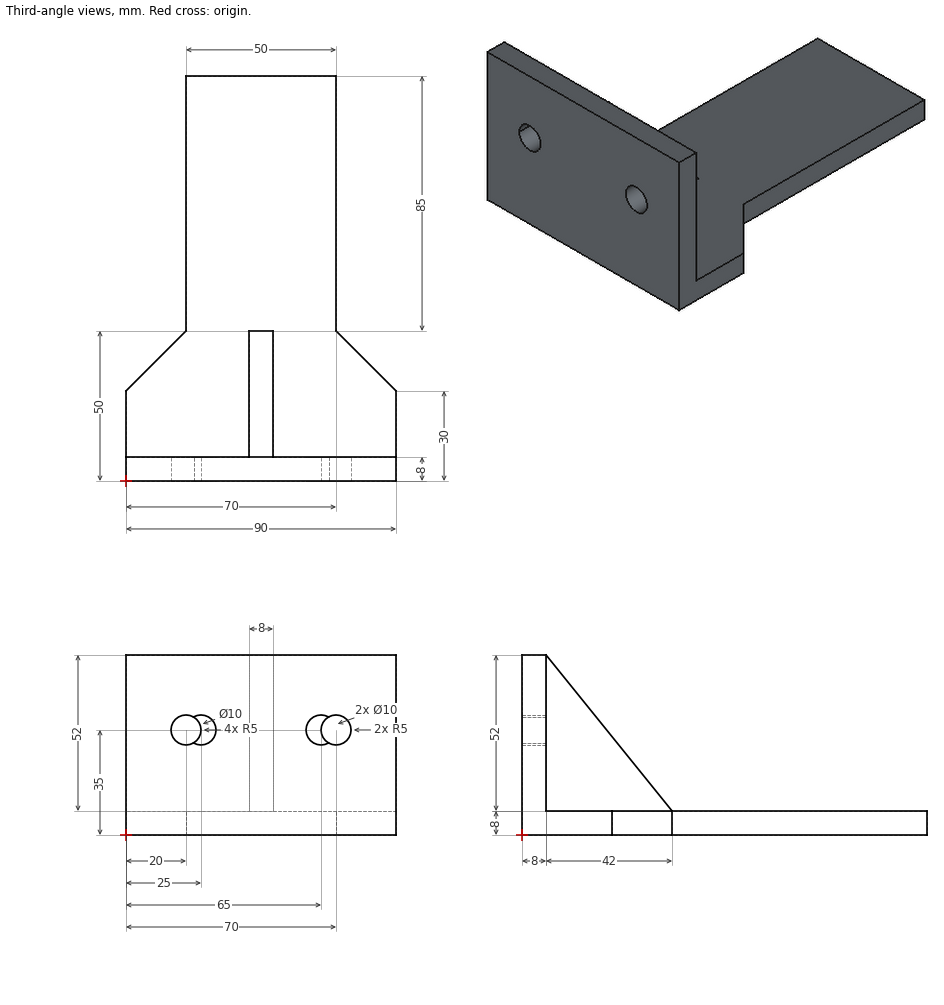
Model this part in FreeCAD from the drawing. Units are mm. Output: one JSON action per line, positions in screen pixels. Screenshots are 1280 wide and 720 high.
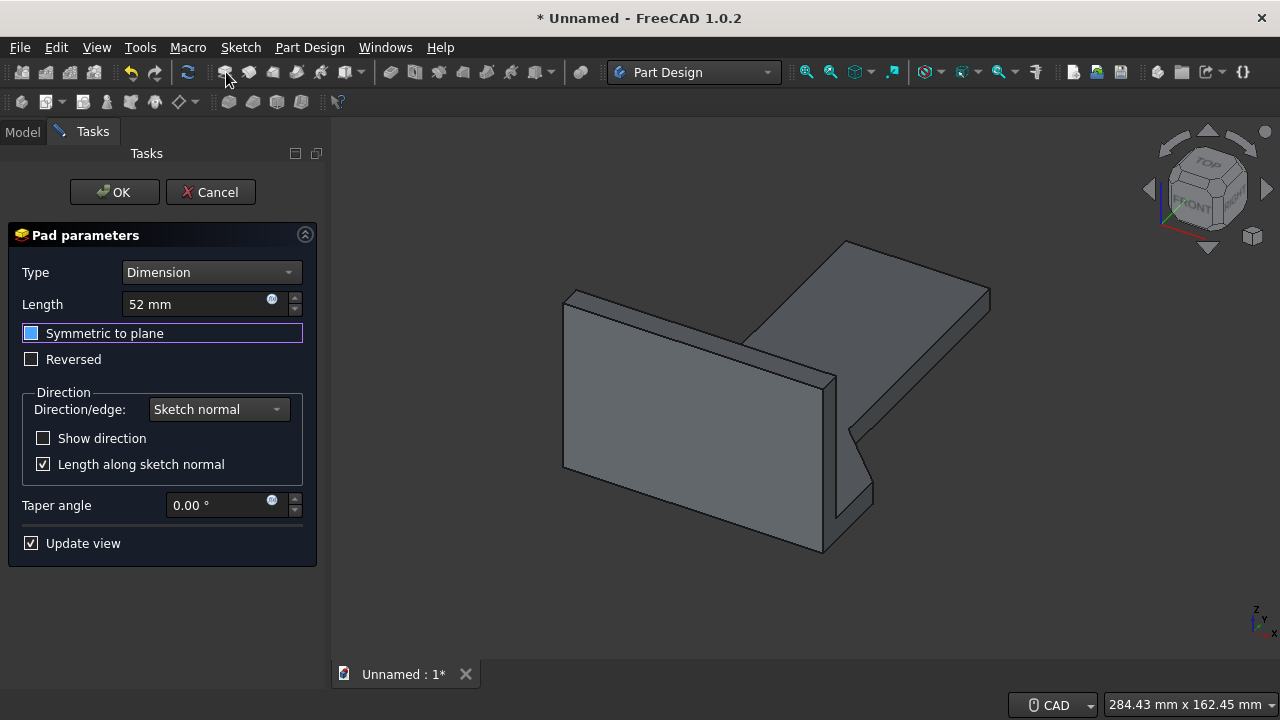
{"action": "left_click", "coordinate": [115, 192]}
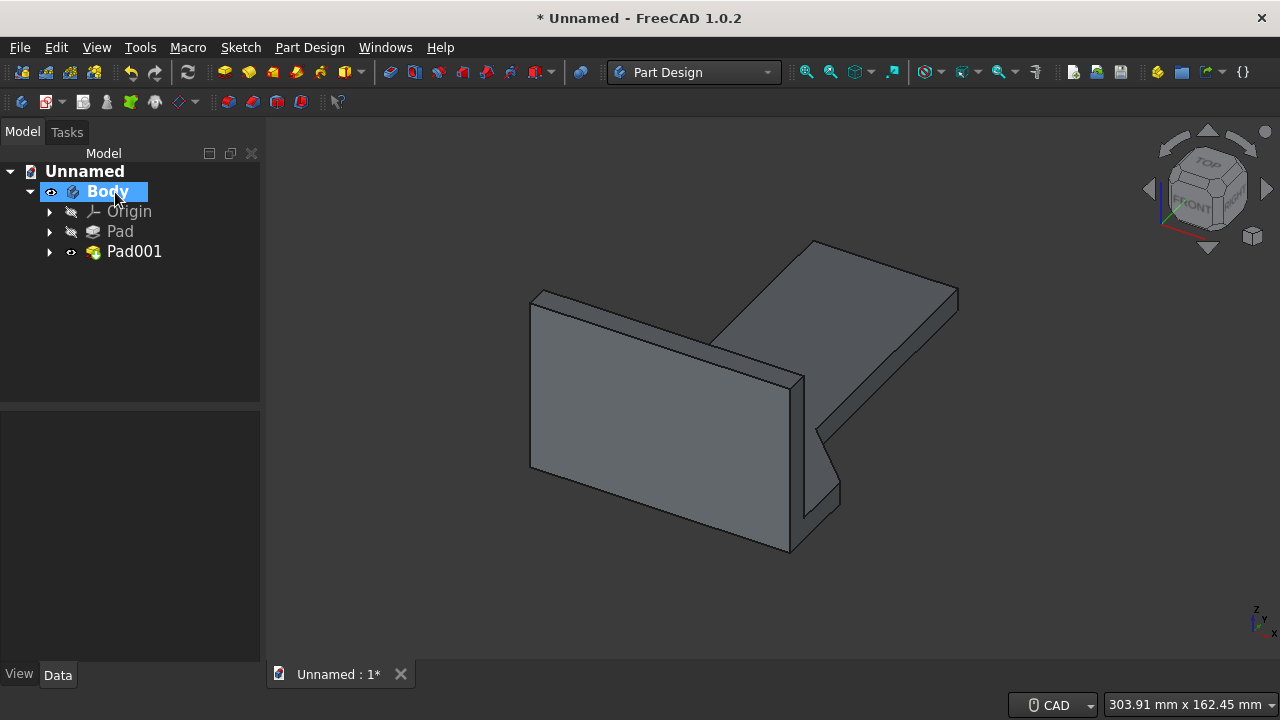
{"action": "left_click", "coordinate": [808, 72]}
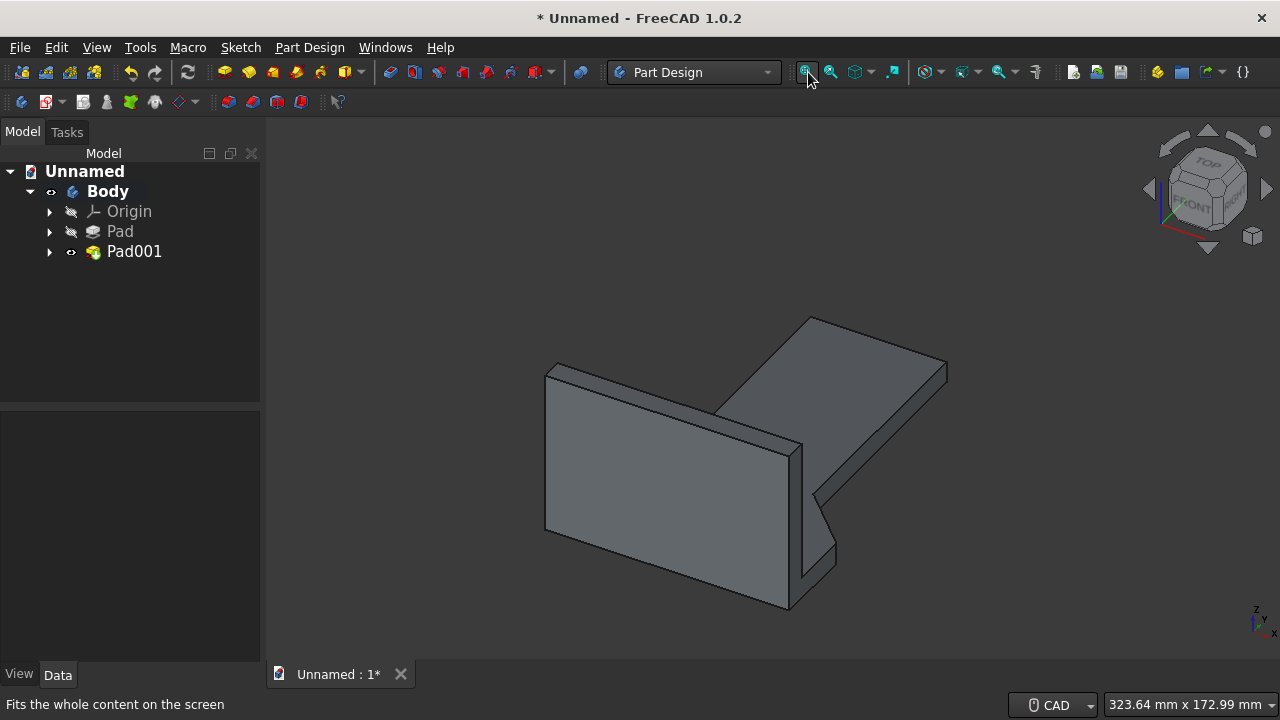
{"action": "left_click", "coordinate": [50, 212]}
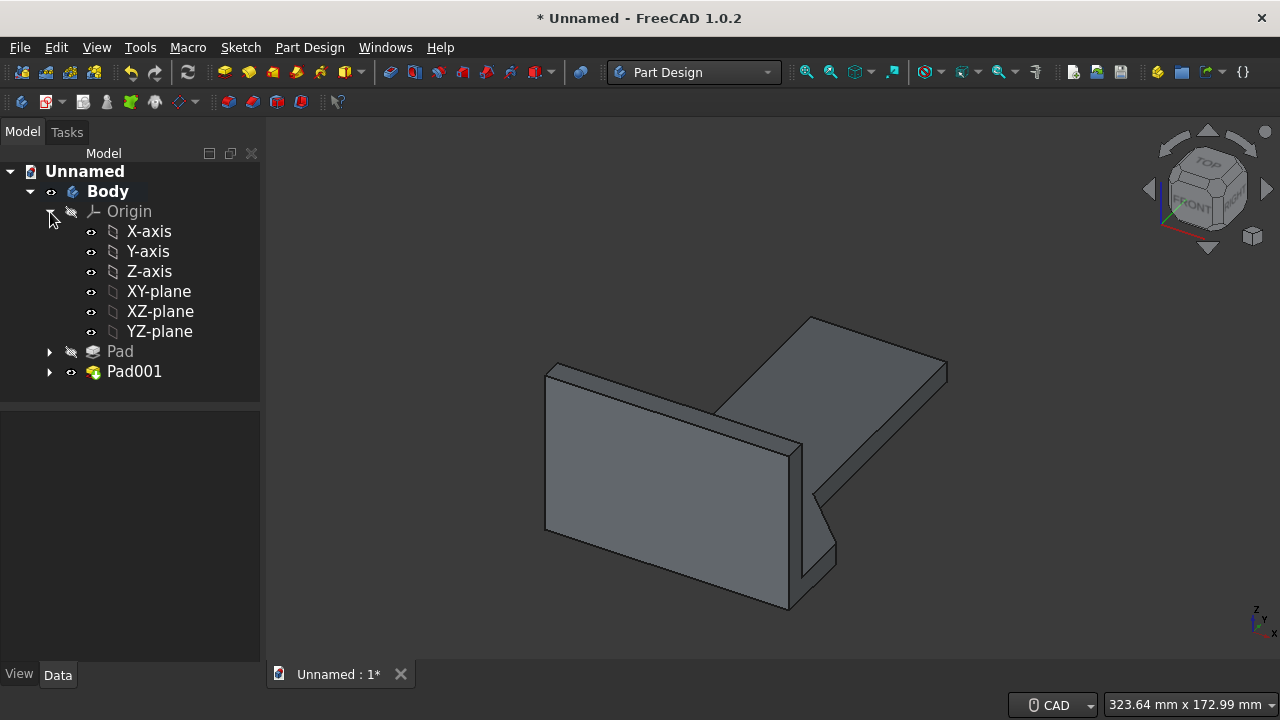
{"action": "left_click", "coordinate": [136, 332]}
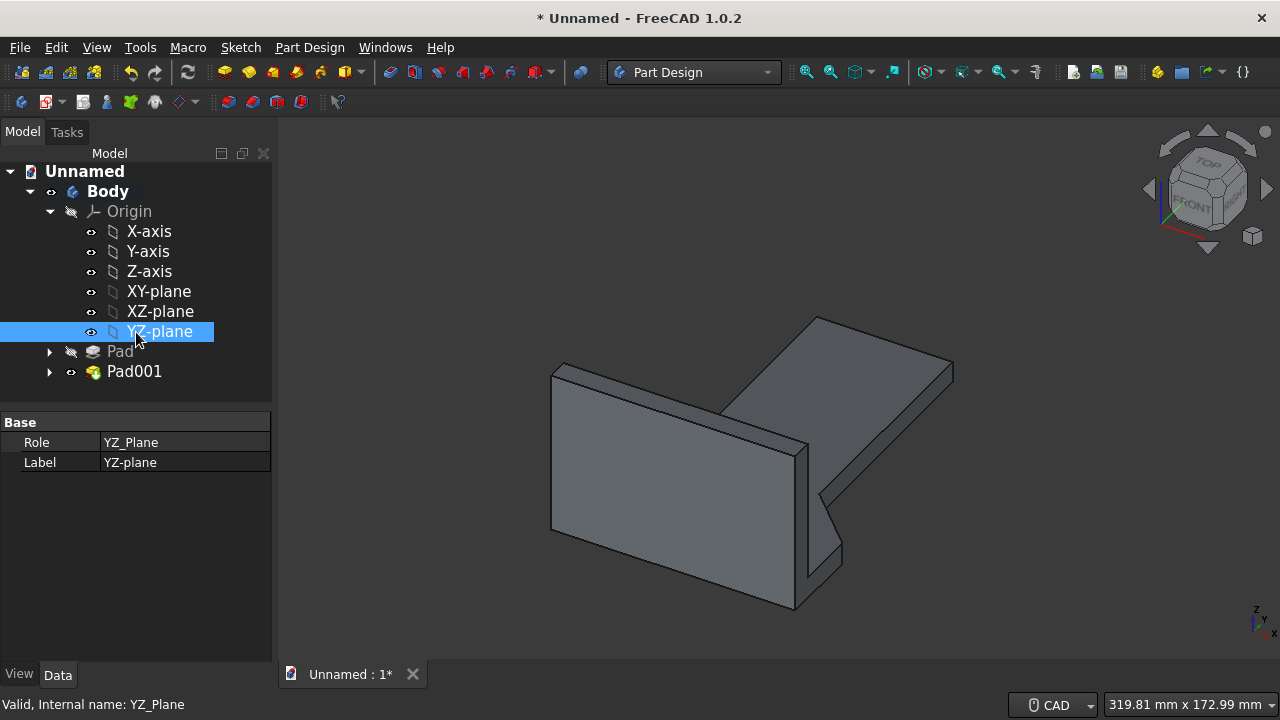
{"action": "left_click", "coordinate": [180, 102]}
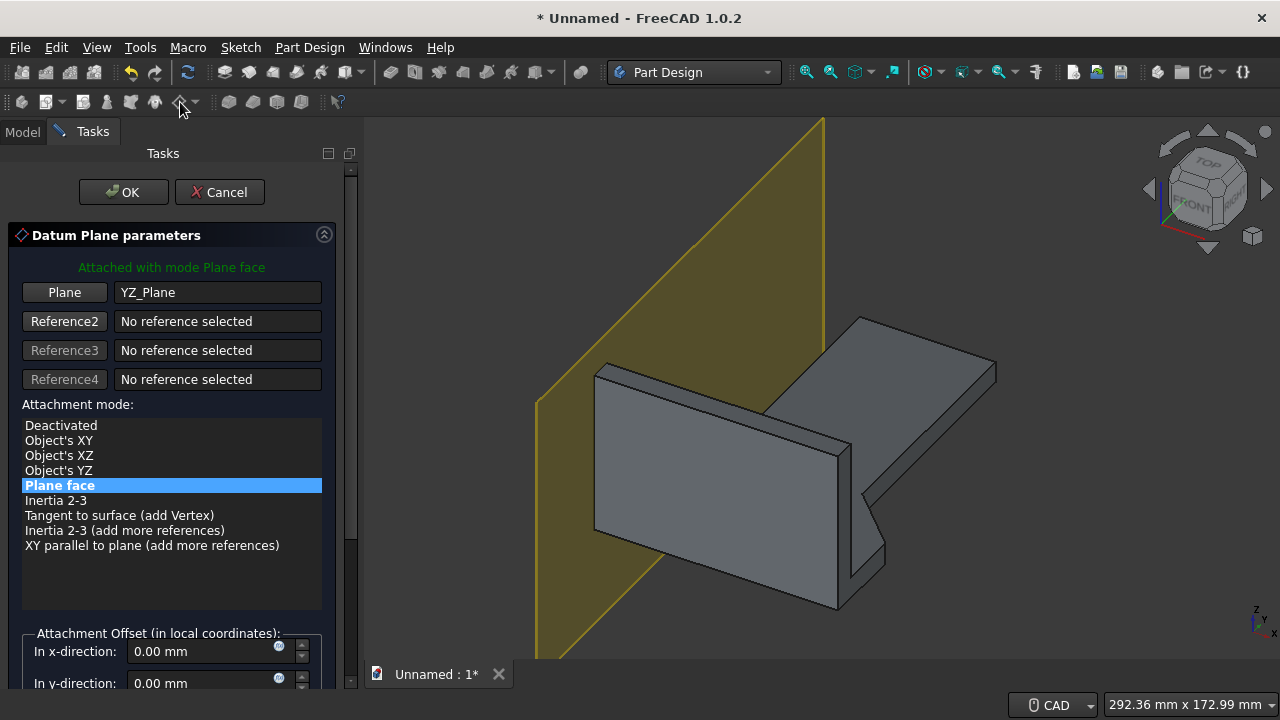
{"action": "scroll", "coordinate": [351, 426], "scroll_direction": "down", "scroll_amount": 2}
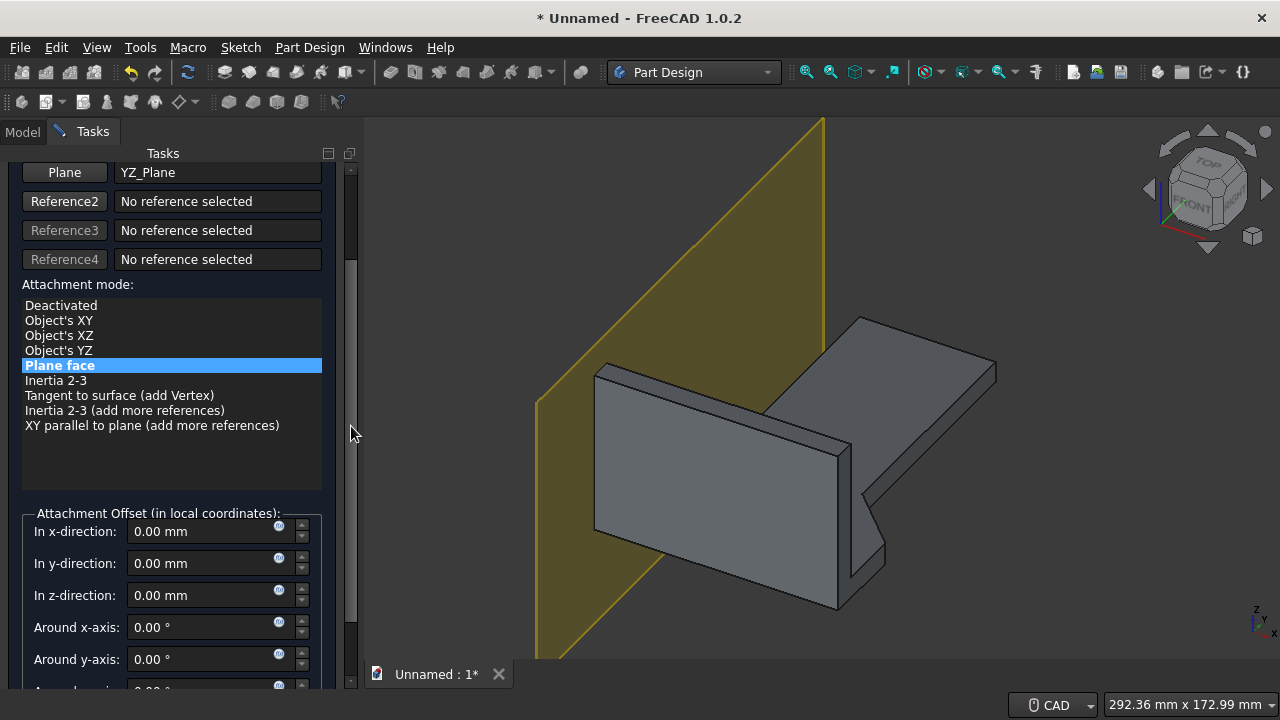
{"action": "triple_click", "coordinate": [210, 595]}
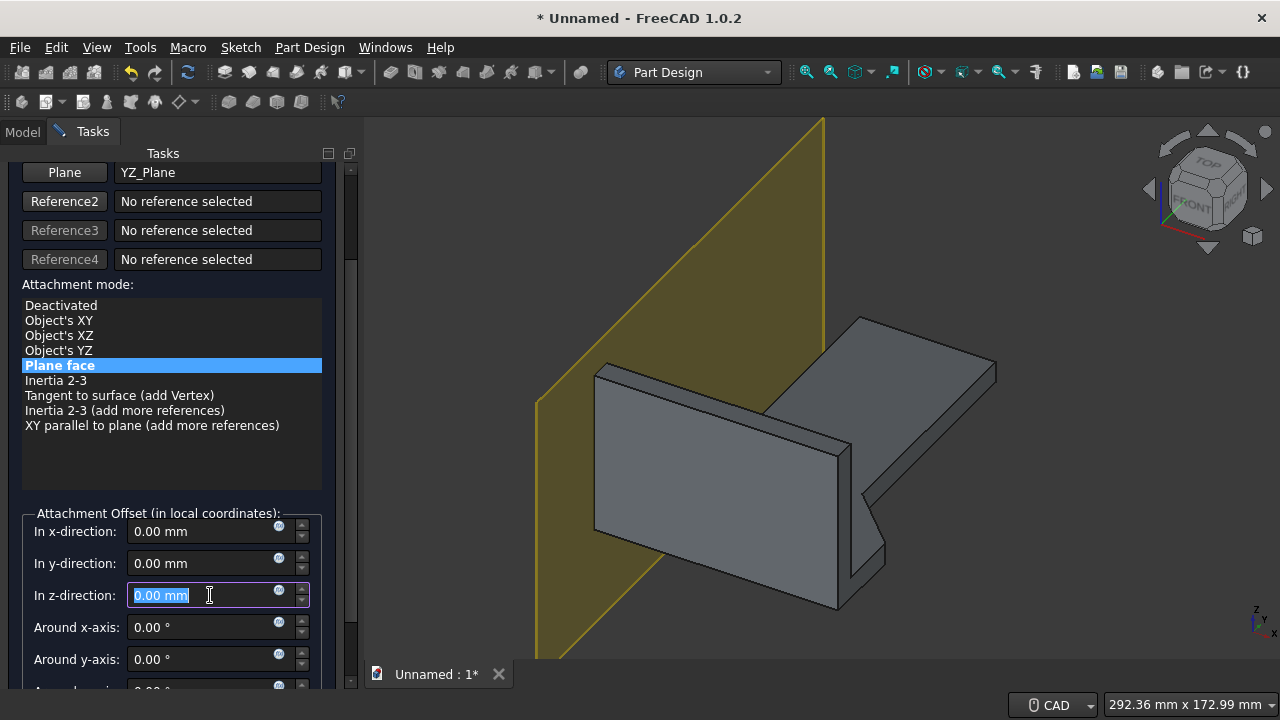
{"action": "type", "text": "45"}
{"action": "key", "text": "Tab"}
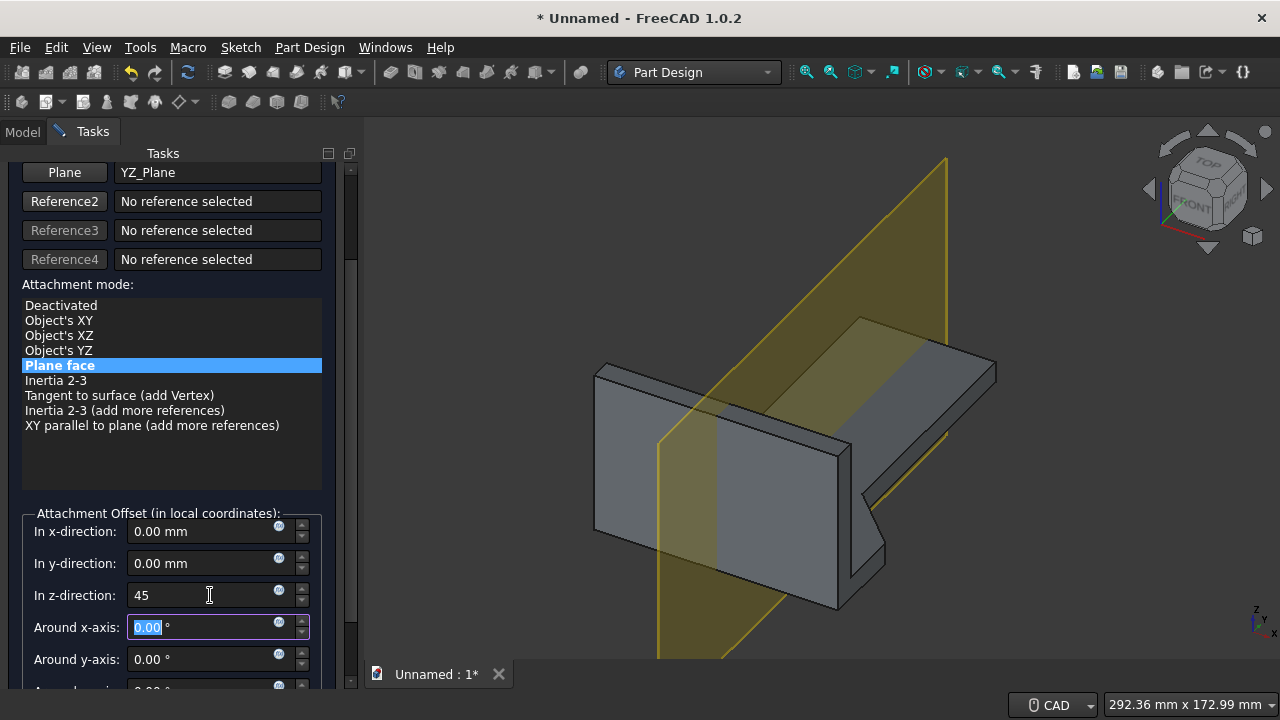
{"action": "scroll", "coordinate": [351, 426], "scroll_direction": "up", "scroll_amount": 3}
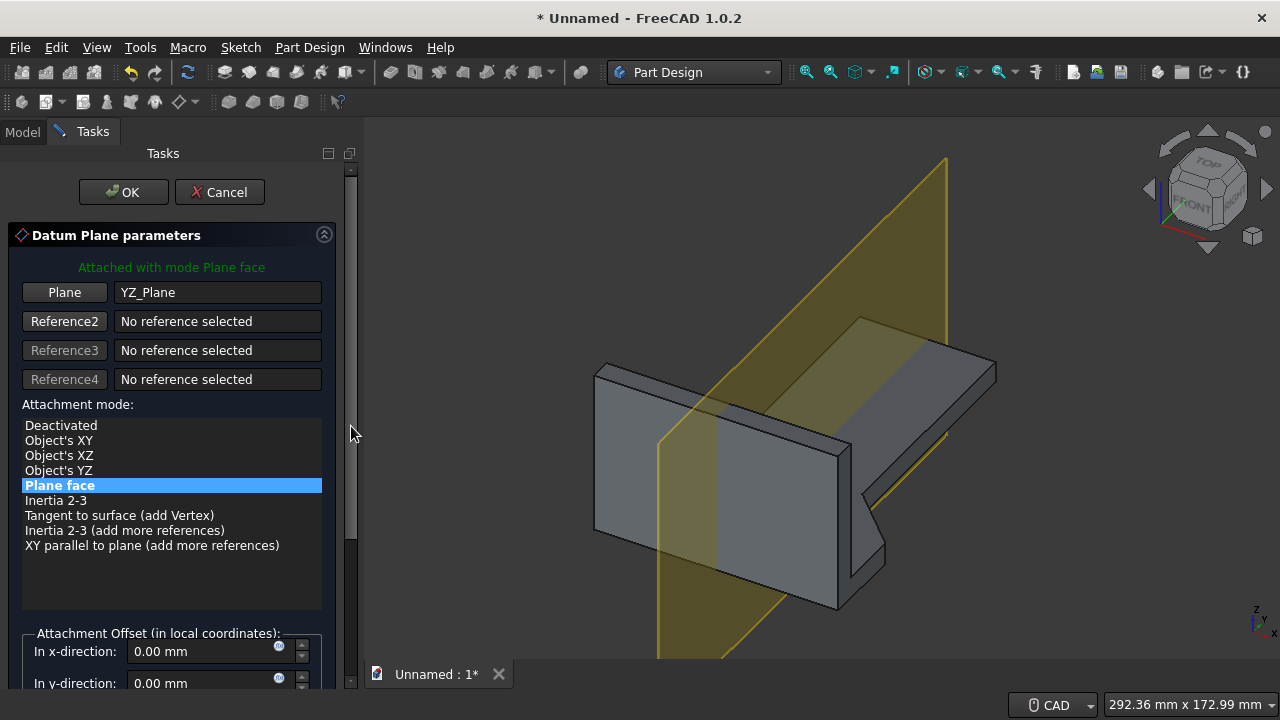
{"action": "left_click", "coordinate": [124, 192]}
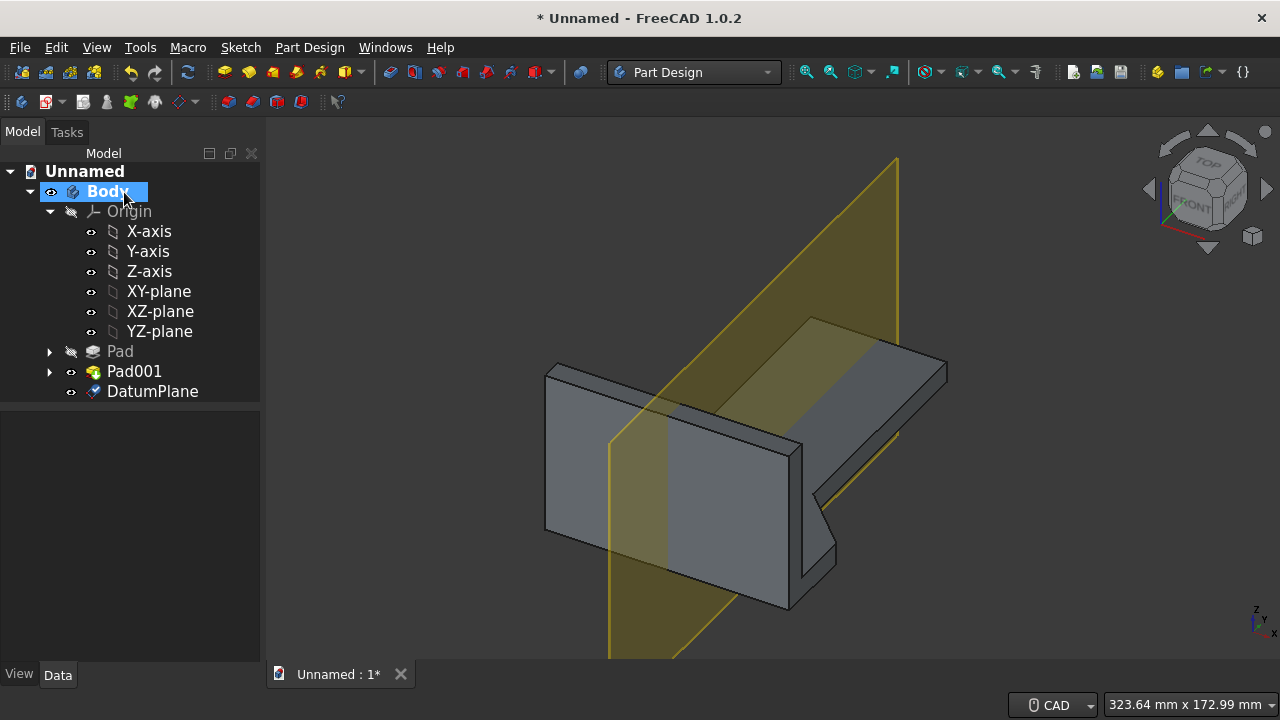
{"action": "left_click", "coordinate": [116, 392]}